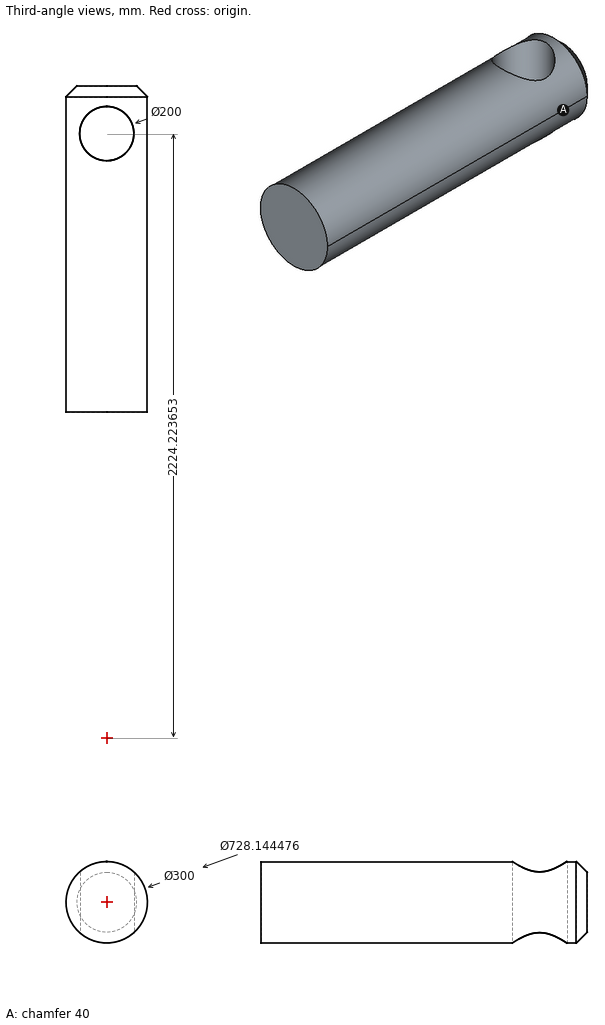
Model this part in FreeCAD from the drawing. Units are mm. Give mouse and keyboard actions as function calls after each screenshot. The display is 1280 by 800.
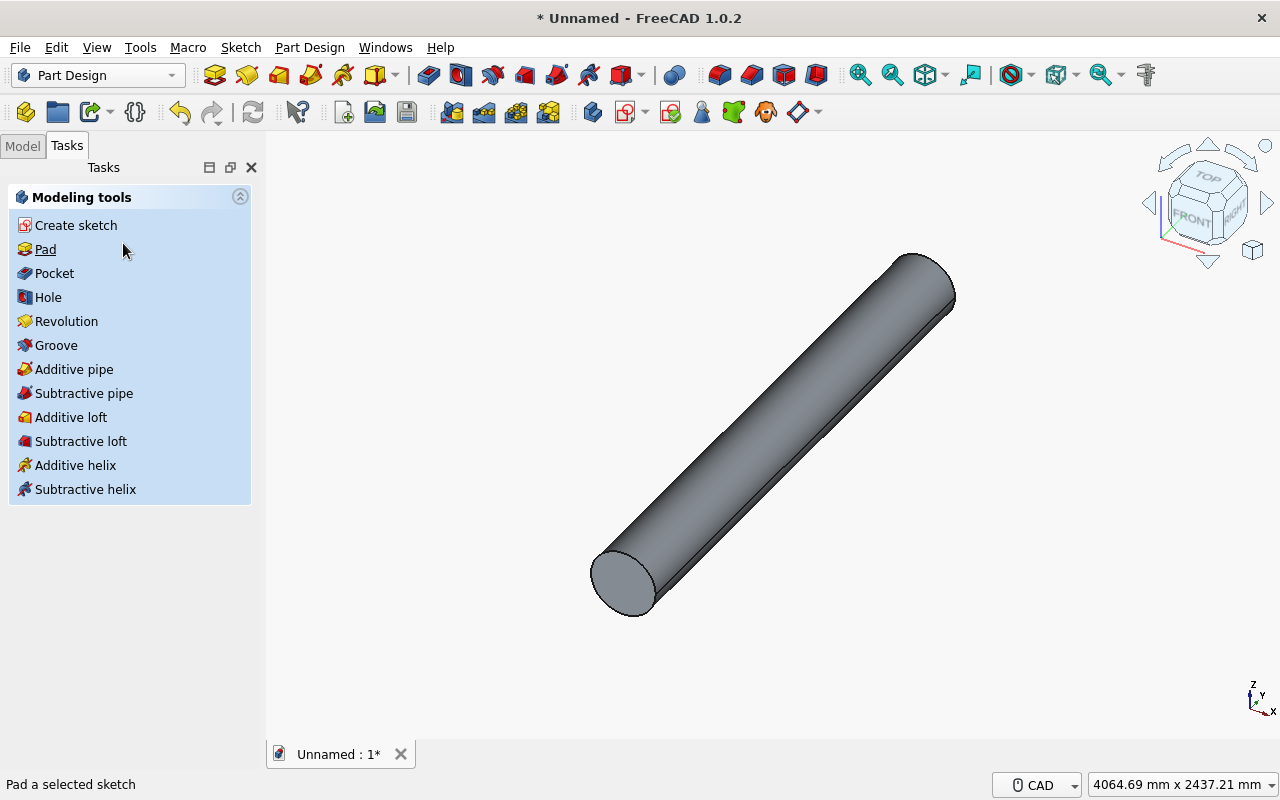
click(430, 76)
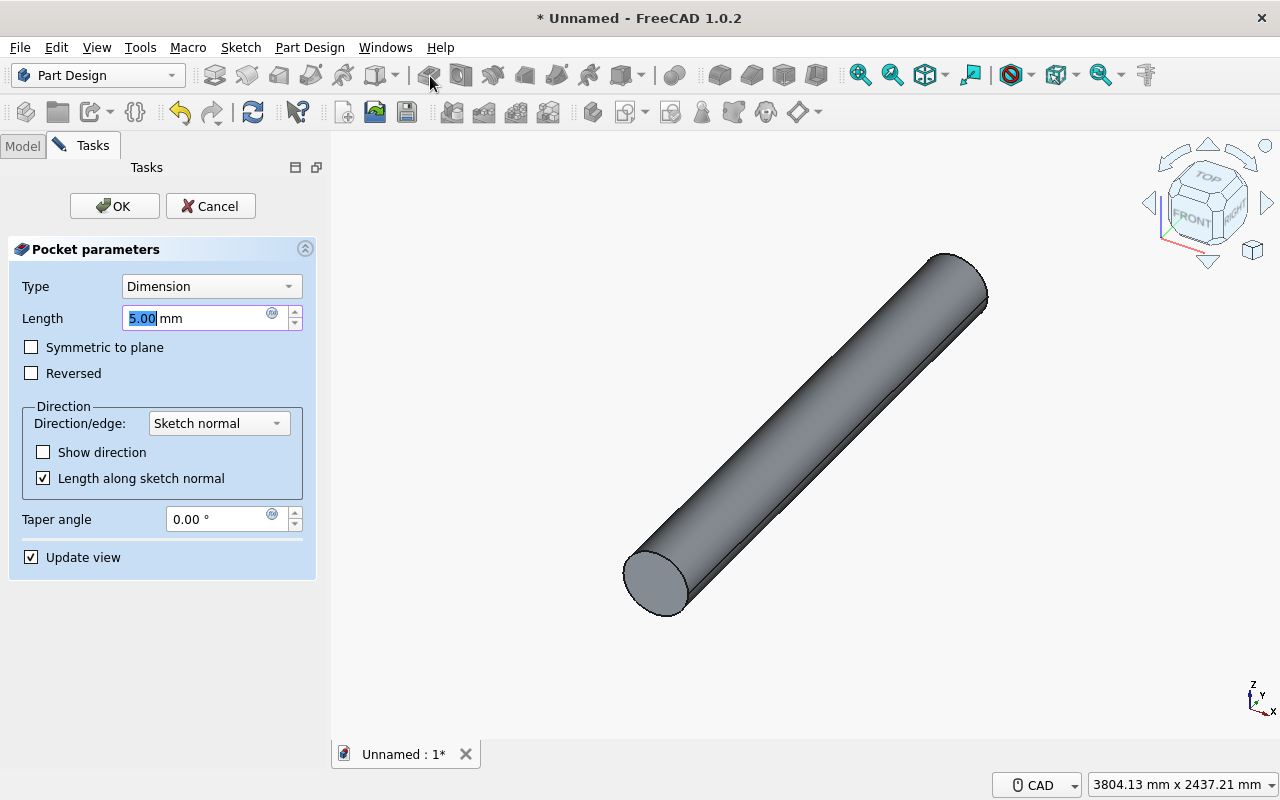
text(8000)
key(Tab)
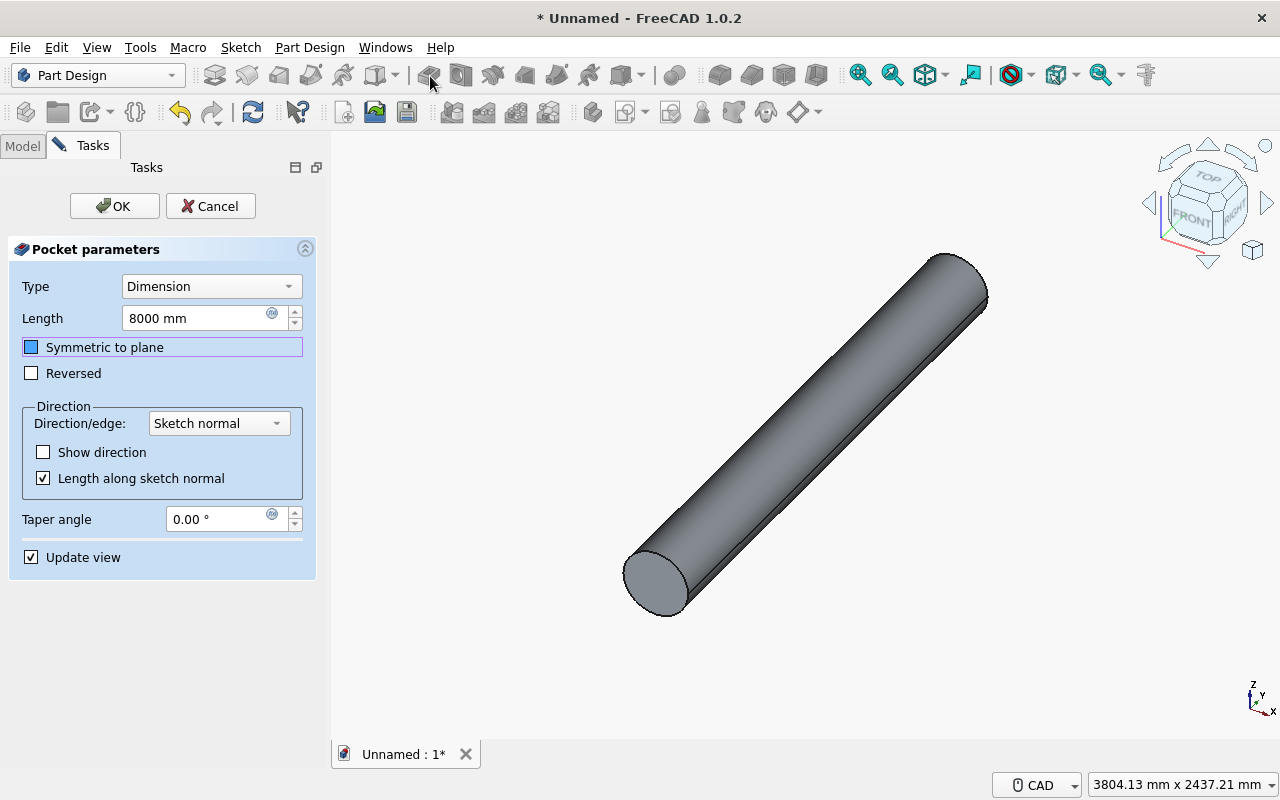
click(30, 347)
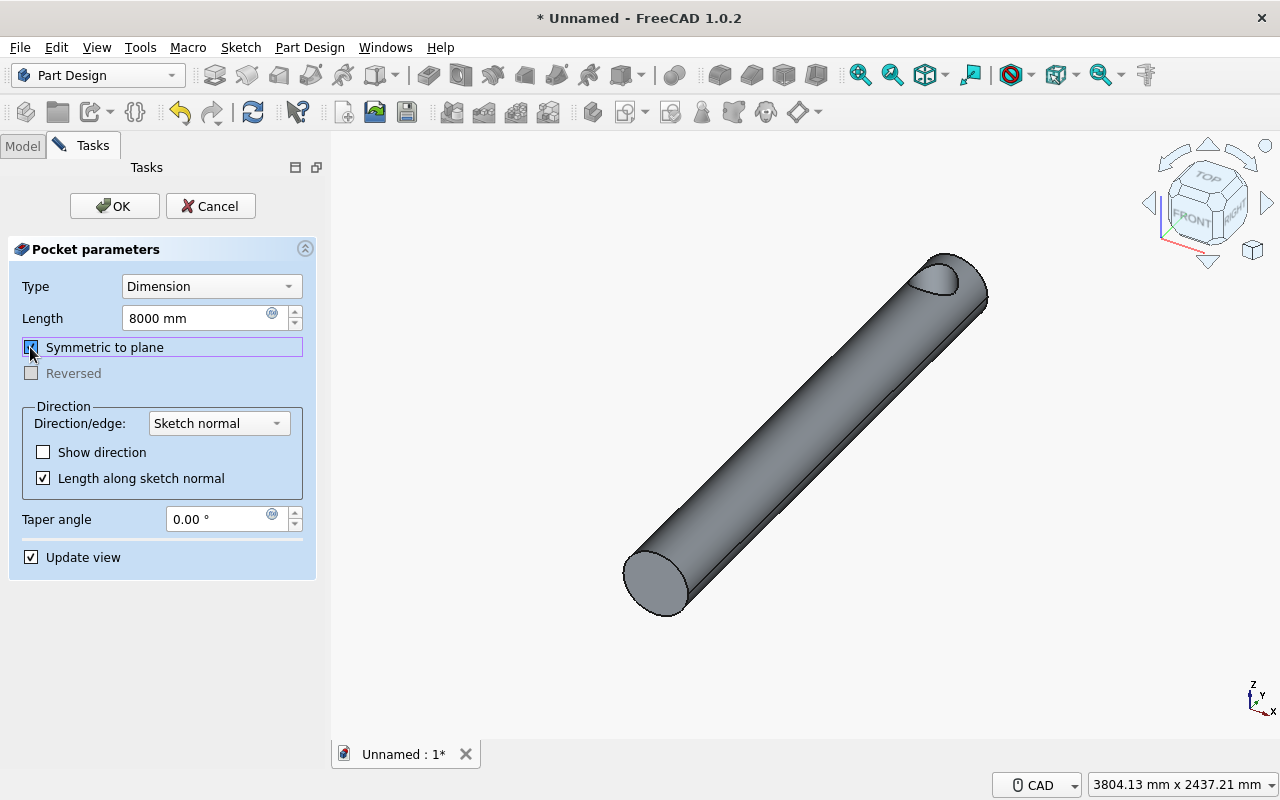
click(115, 206)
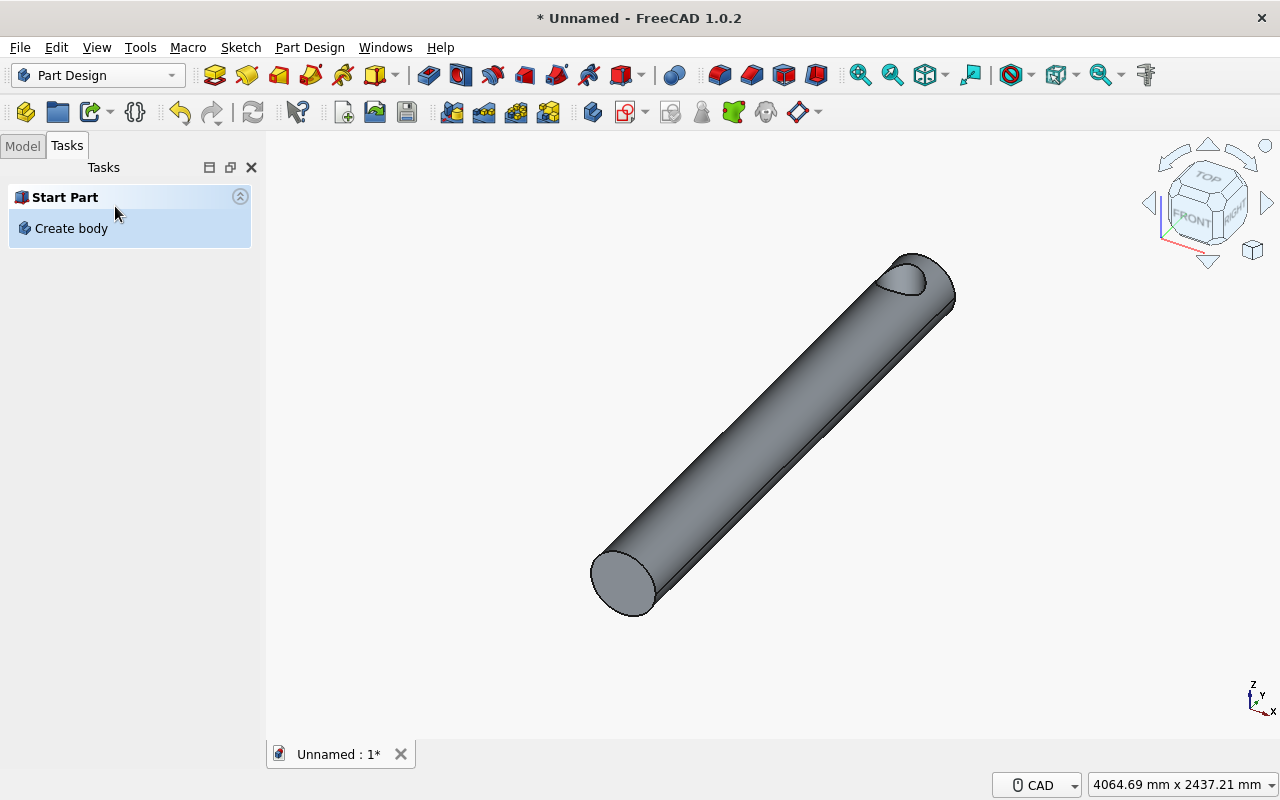
click(623, 583)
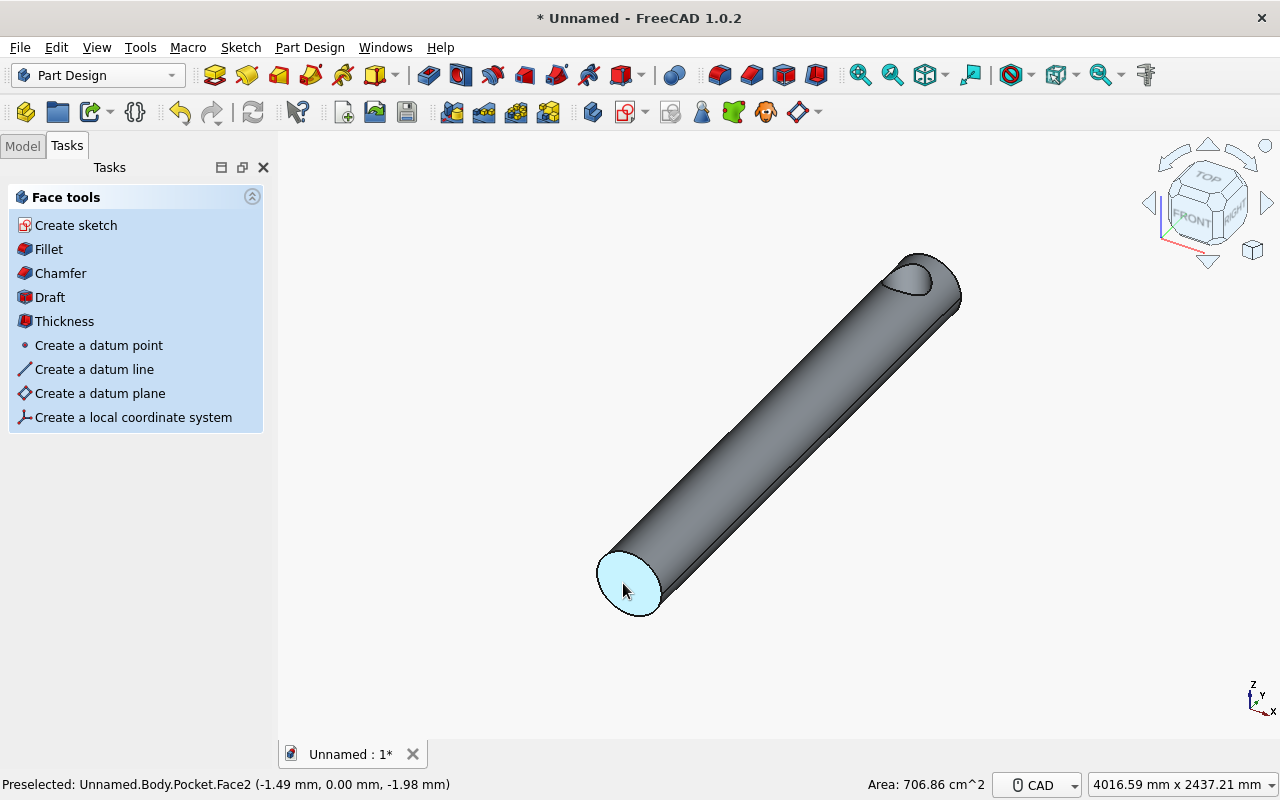
click(626, 112)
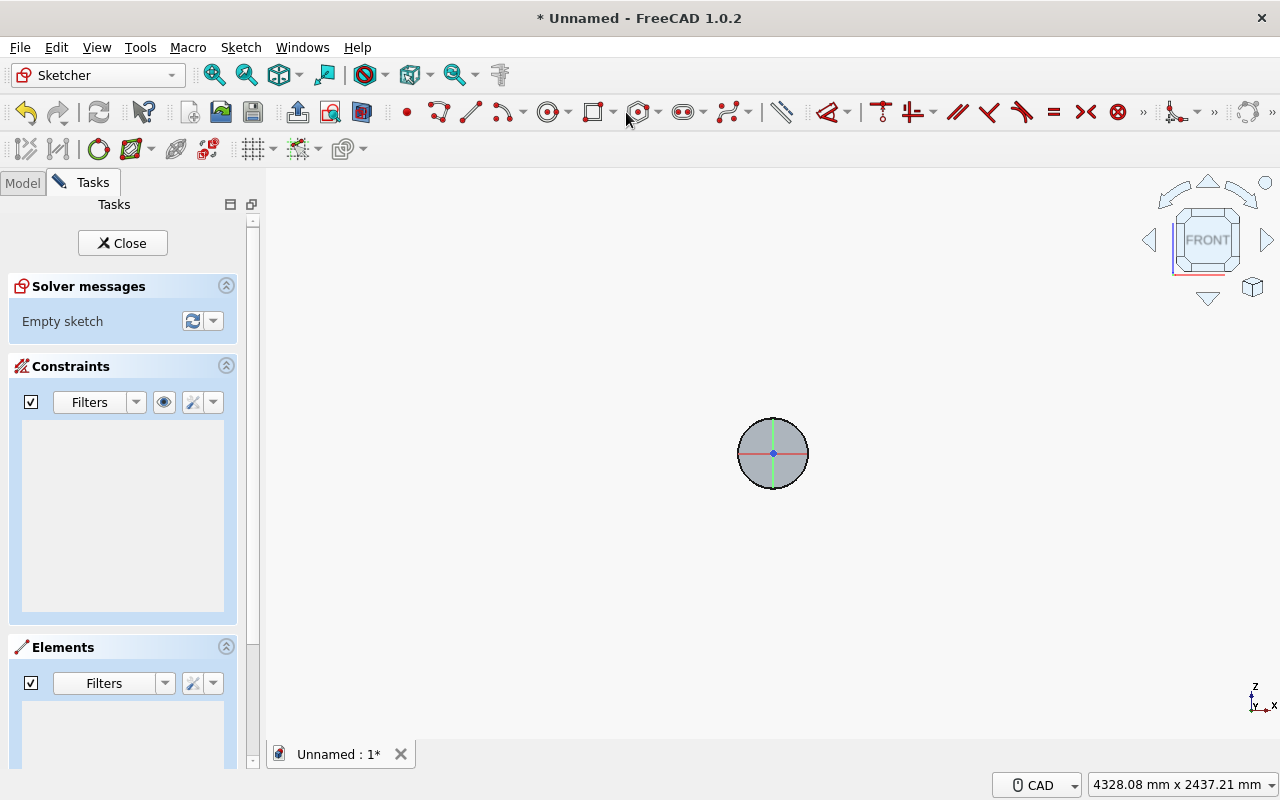
scroll(829, 454, up, 4)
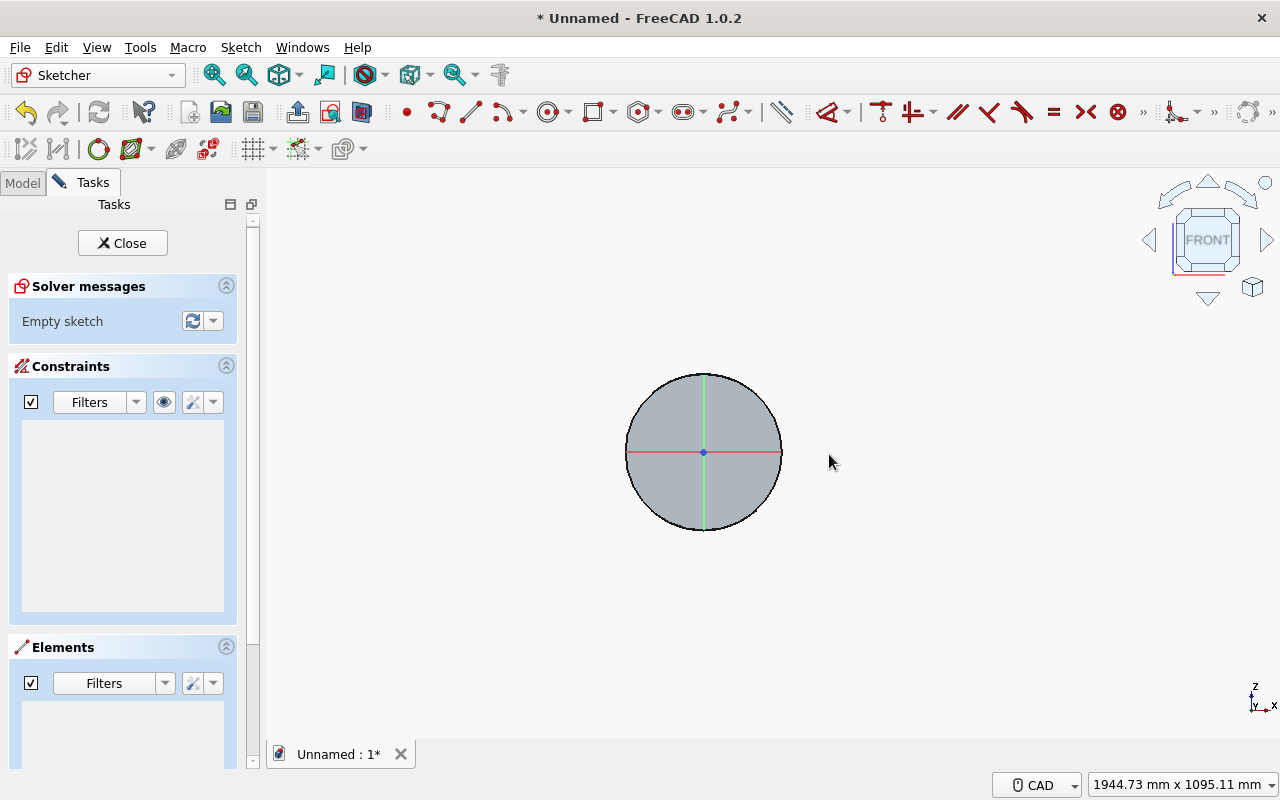
click(548, 112)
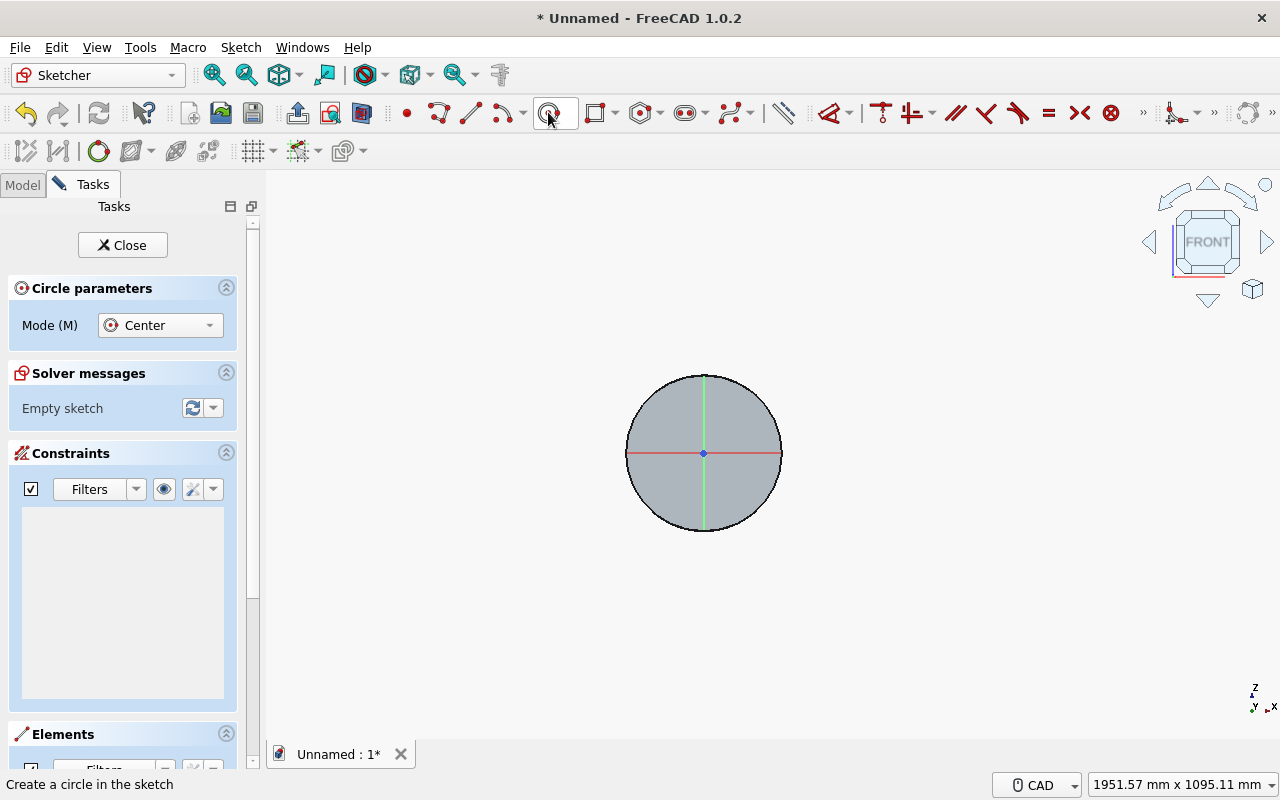
click(704, 453)
move(838, 320)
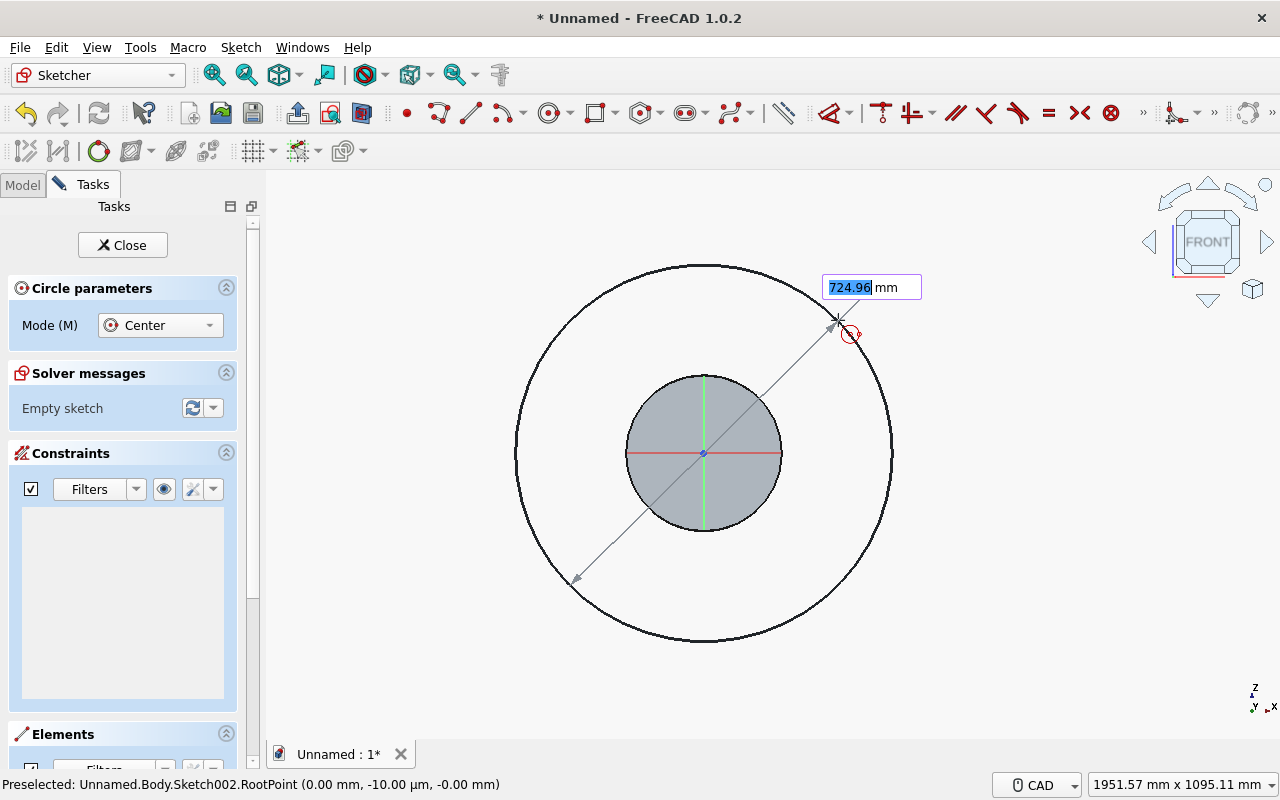
text(728.144476)
key(Return)
key(Escape)